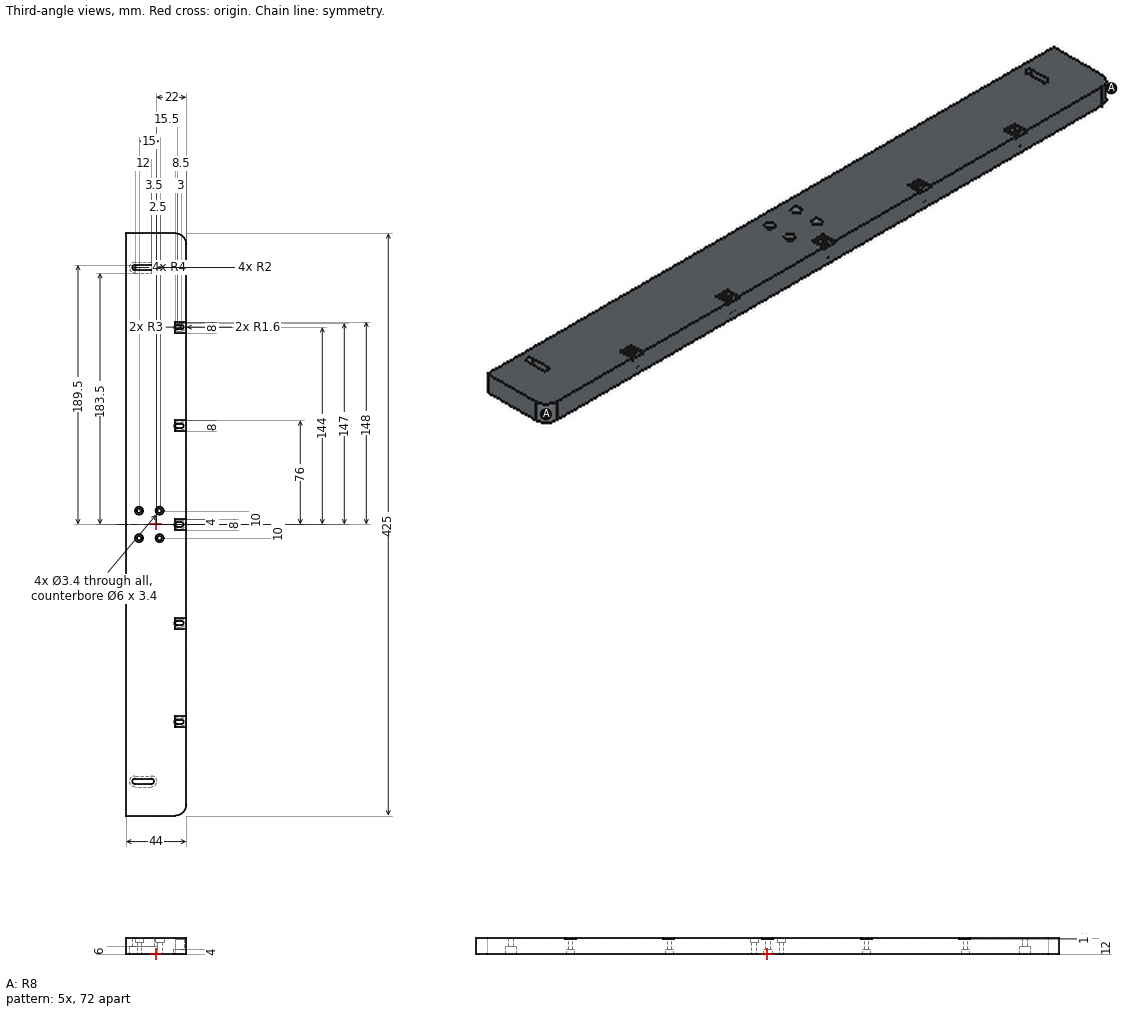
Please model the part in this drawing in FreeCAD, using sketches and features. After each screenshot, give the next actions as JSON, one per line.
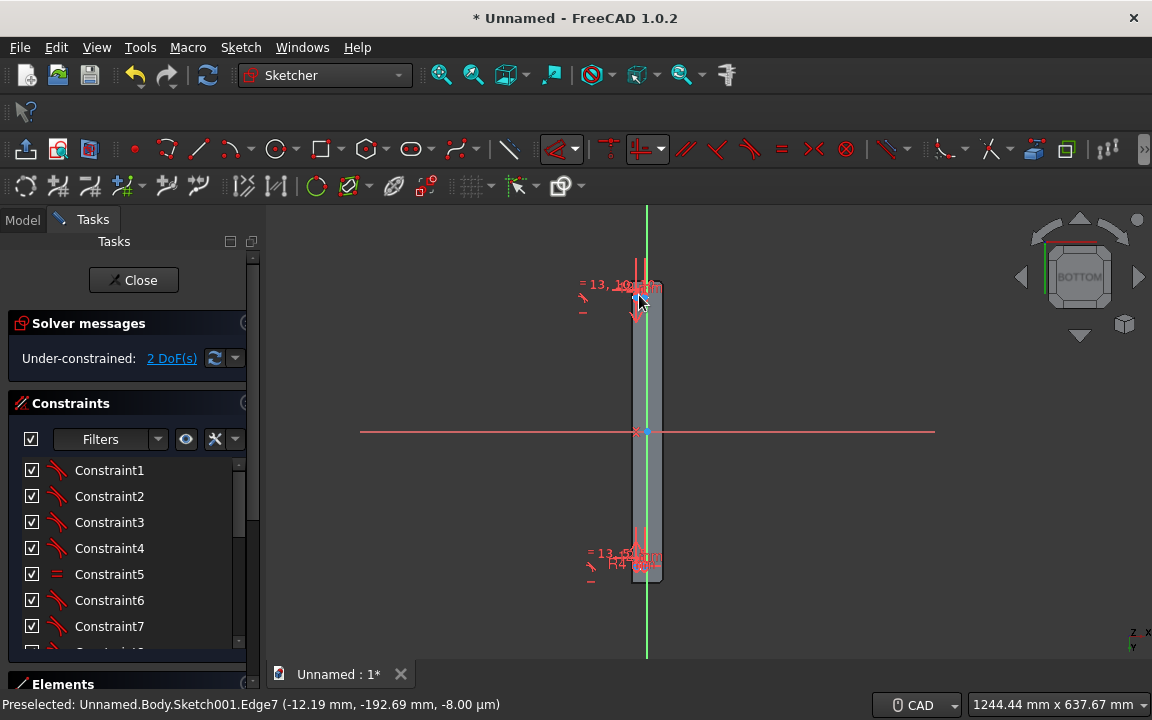
{"action": "scroll", "coordinate": [645, 569], "scroll_direction": "up", "scroll_amount": 14}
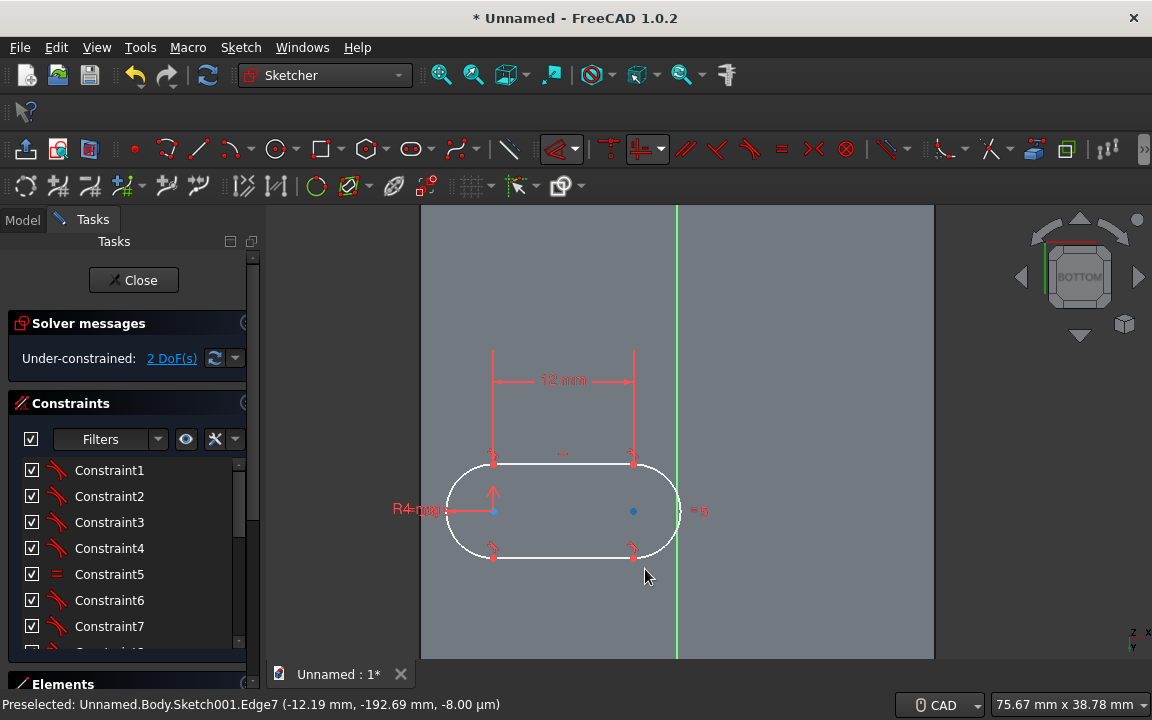
{"action": "left_click", "coordinate": [634, 558]}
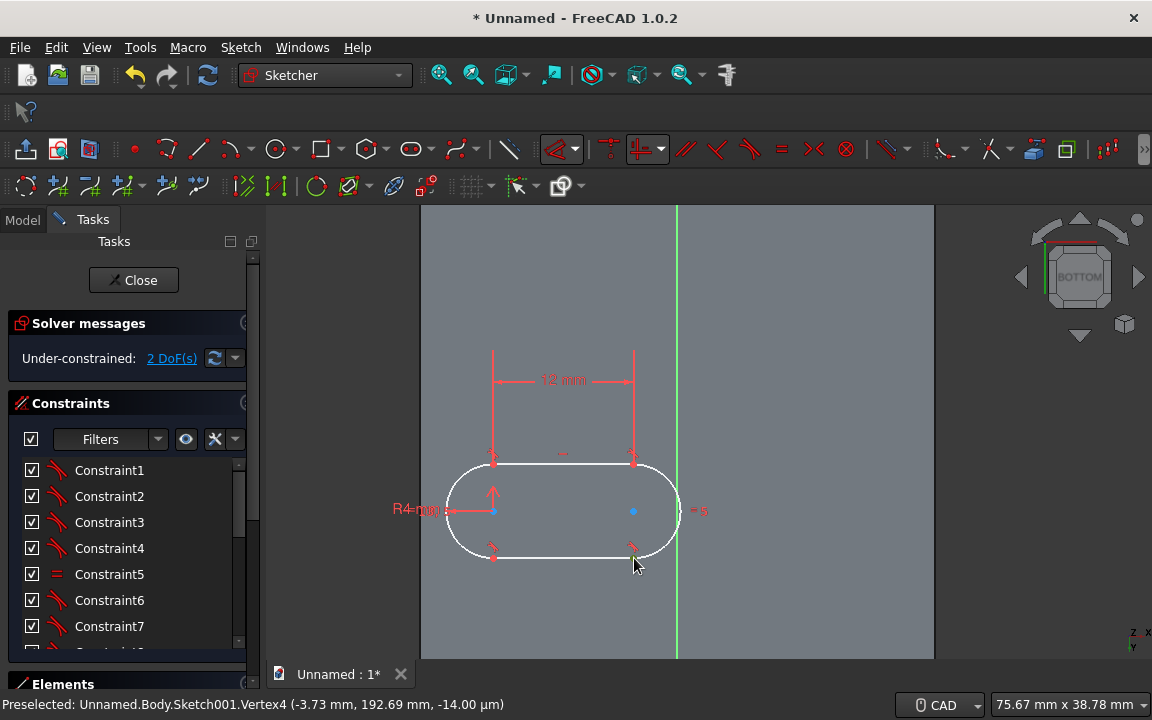
{"action": "key", "text": "l"}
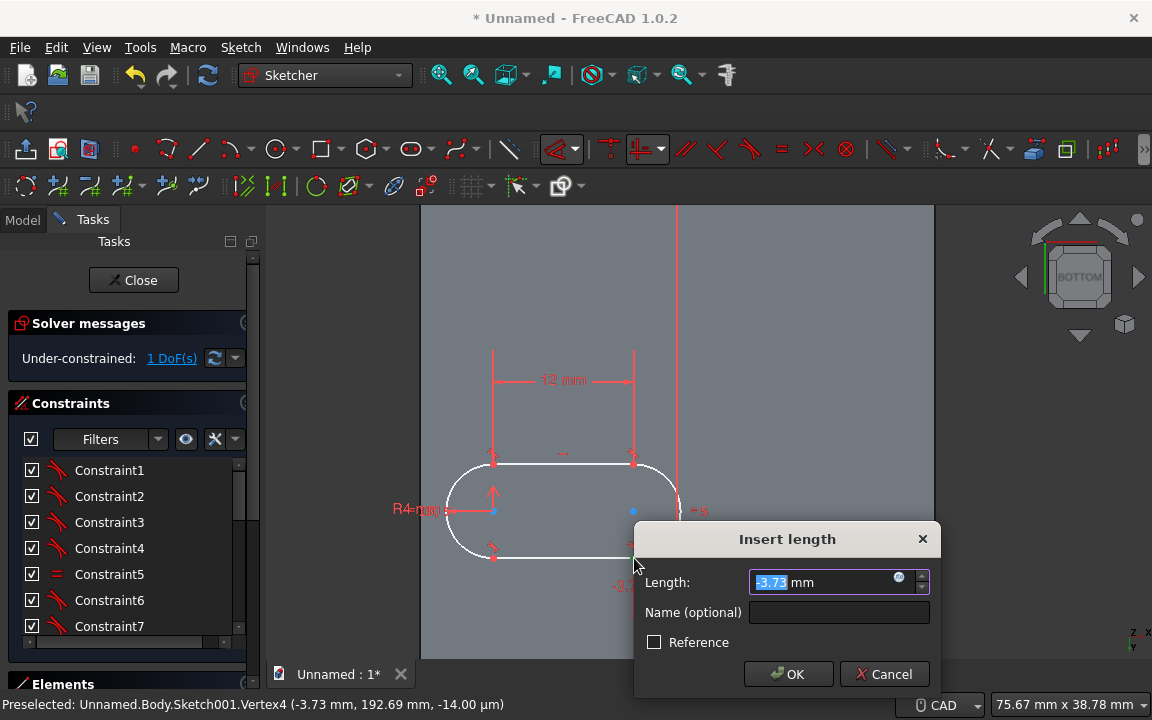
{"action": "type", "text": "-3.5"}
{"action": "key", "text": "Return"}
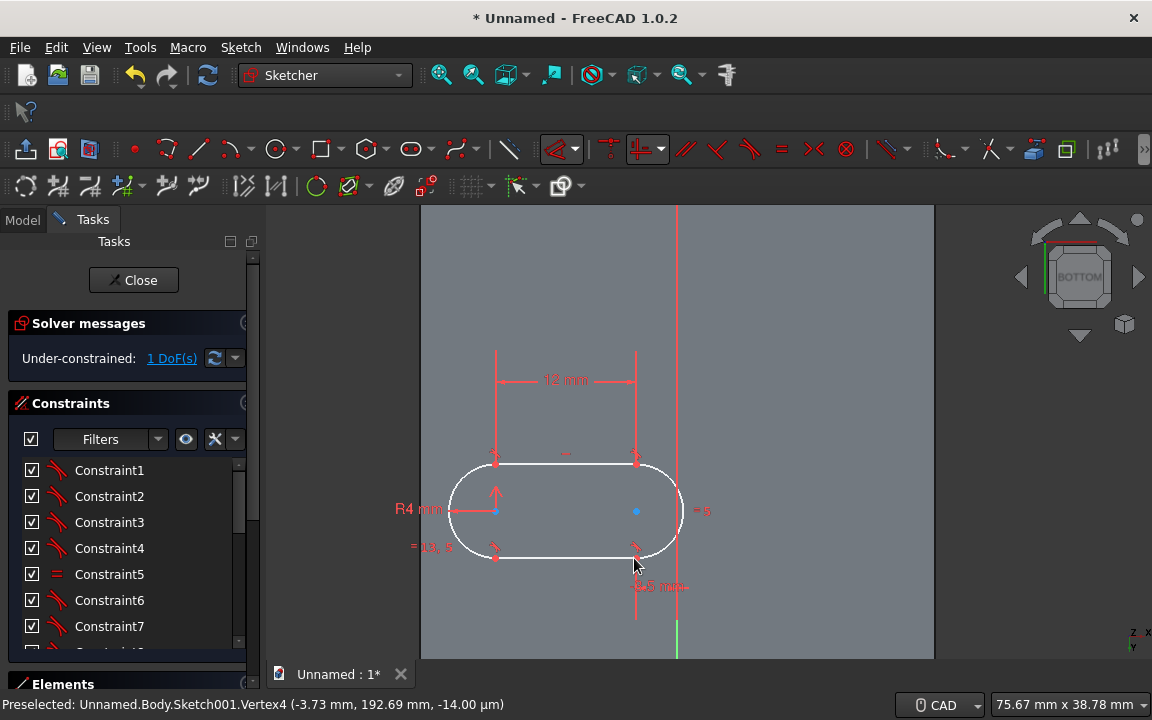
{"action": "scroll", "coordinate": [645, 570], "scroll_direction": "down", "scroll_amount": 14}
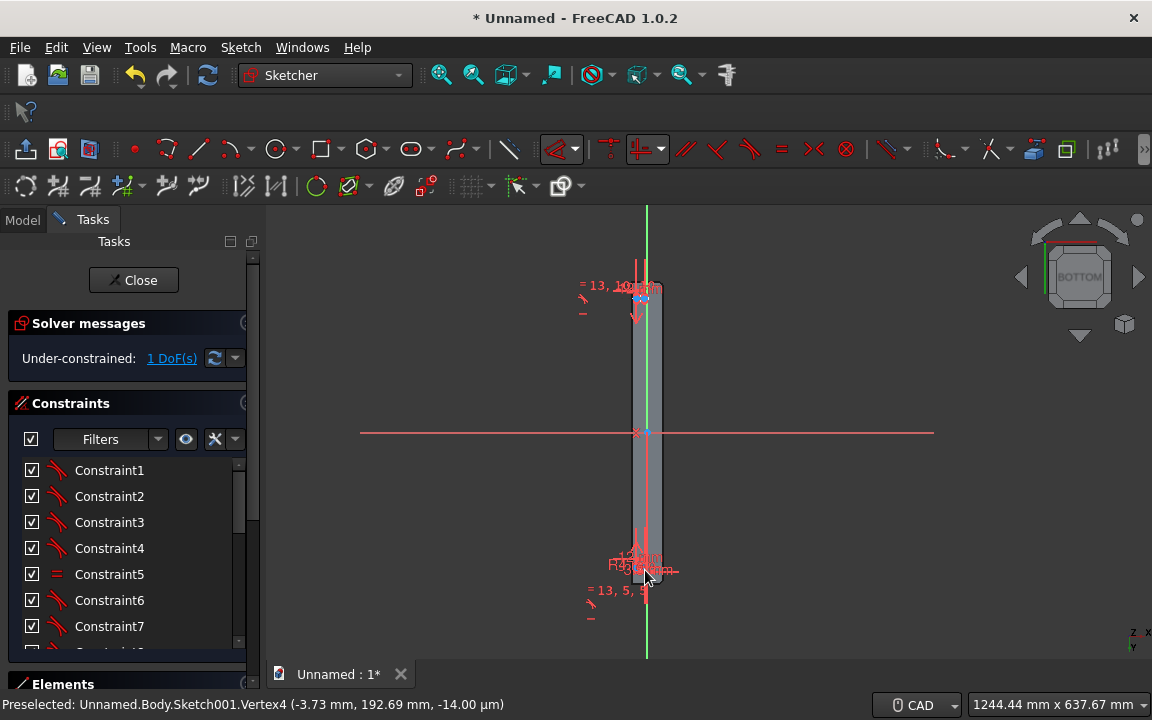
{"action": "scroll", "coordinate": [636, 564], "scroll_direction": "up", "scroll_amount": 8}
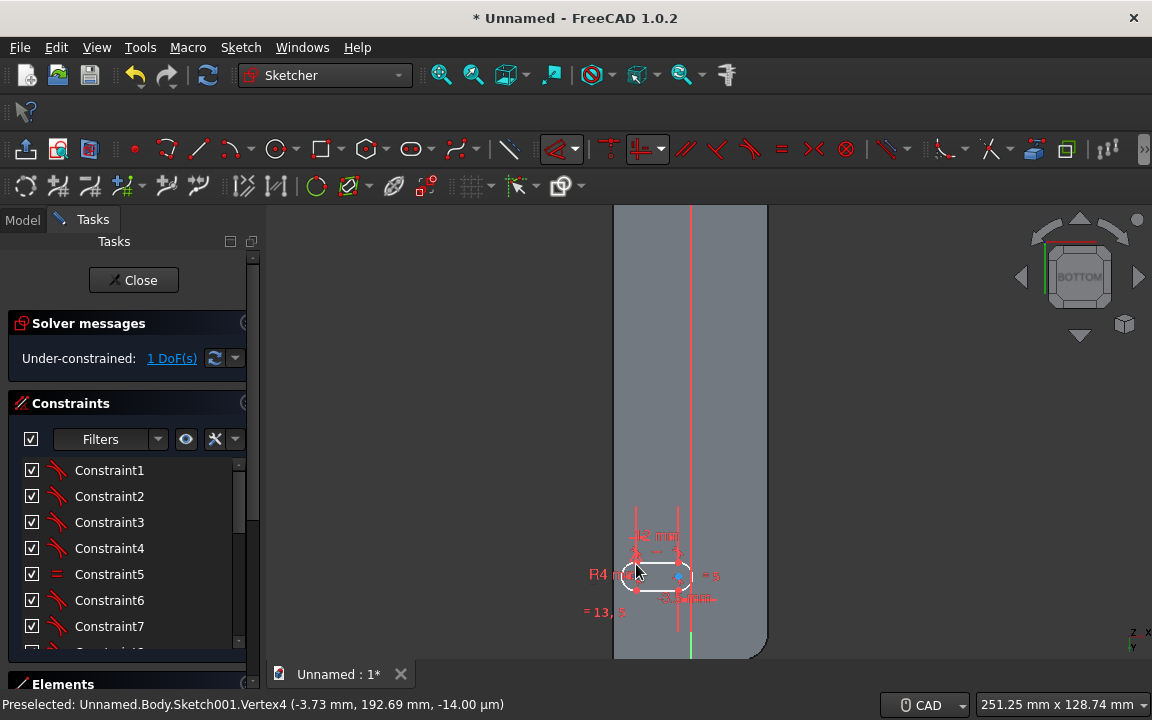
{"action": "left_click", "coordinate": [636, 563]}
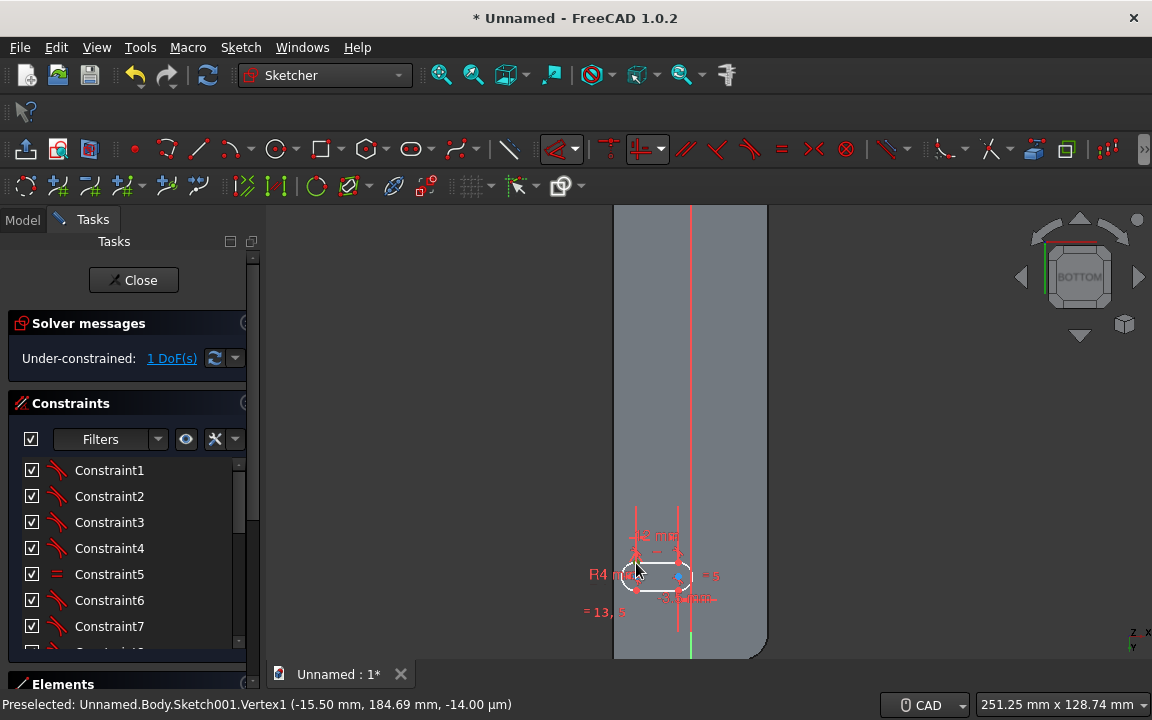
{"action": "left_click", "coordinate": [578, 150]}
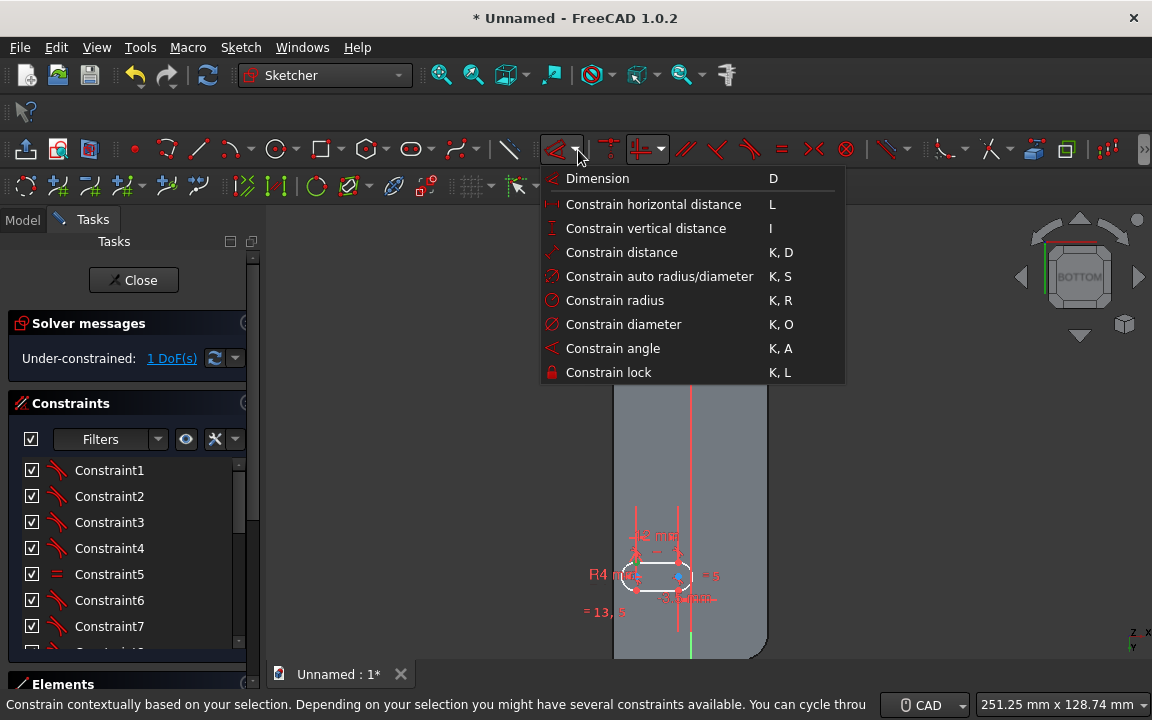
{"action": "left_click", "coordinate": [693, 228]}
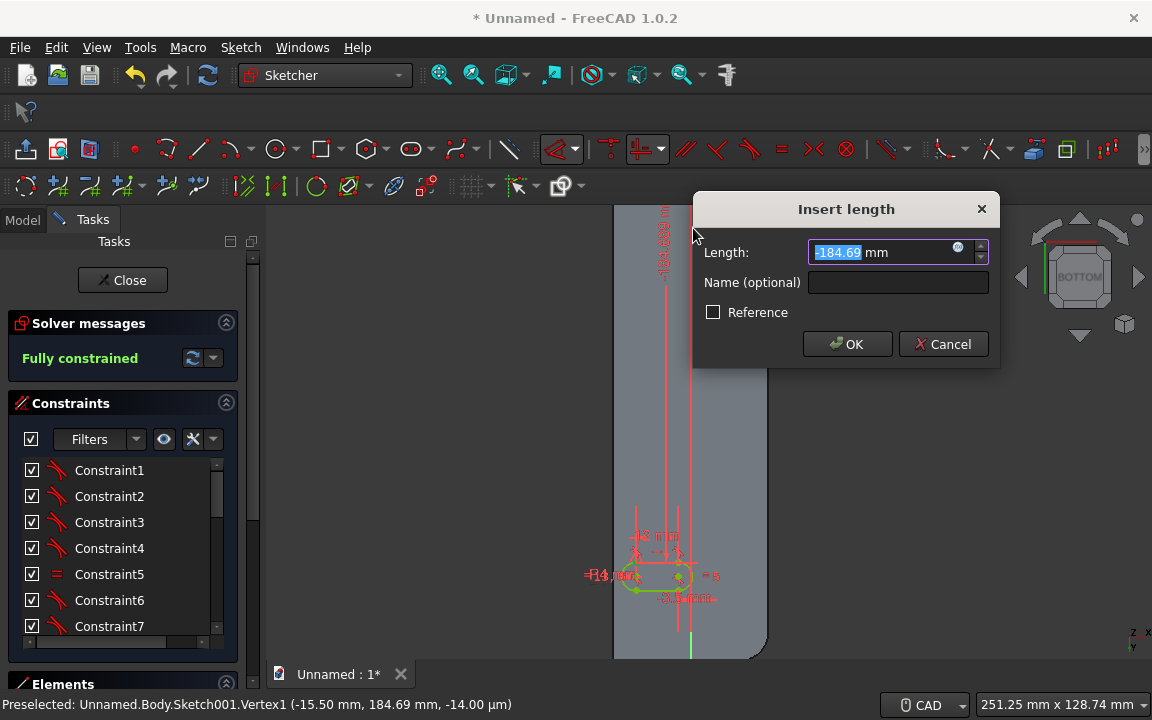
{"action": "type", "text": "-183.5"}
{"action": "key", "text": "Return"}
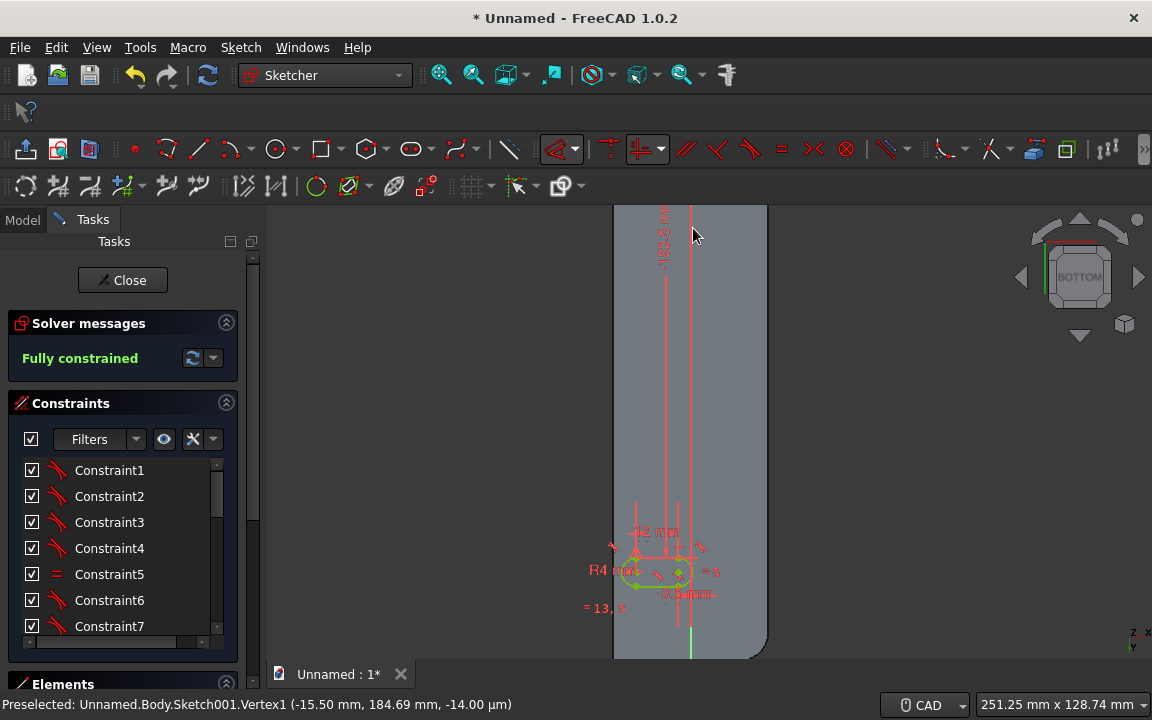
{"action": "left_click", "coordinate": [123, 280]}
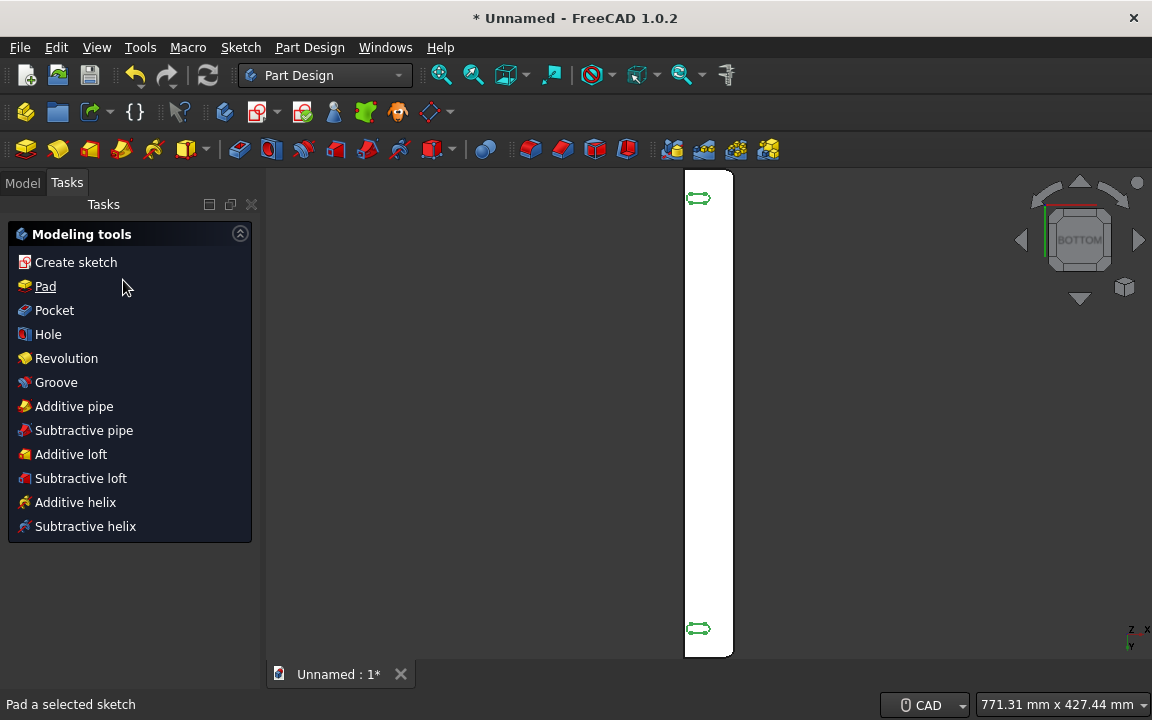
{"action": "left_click", "coordinate": [240, 150]}